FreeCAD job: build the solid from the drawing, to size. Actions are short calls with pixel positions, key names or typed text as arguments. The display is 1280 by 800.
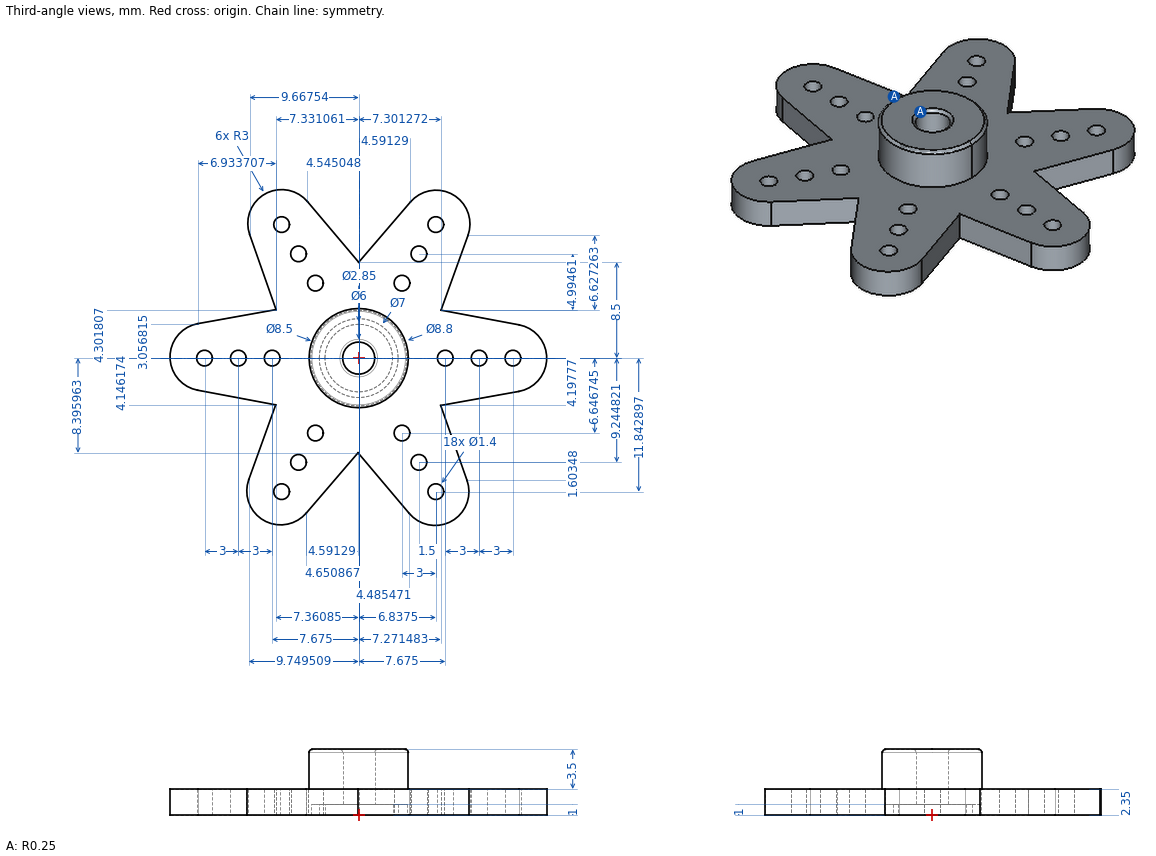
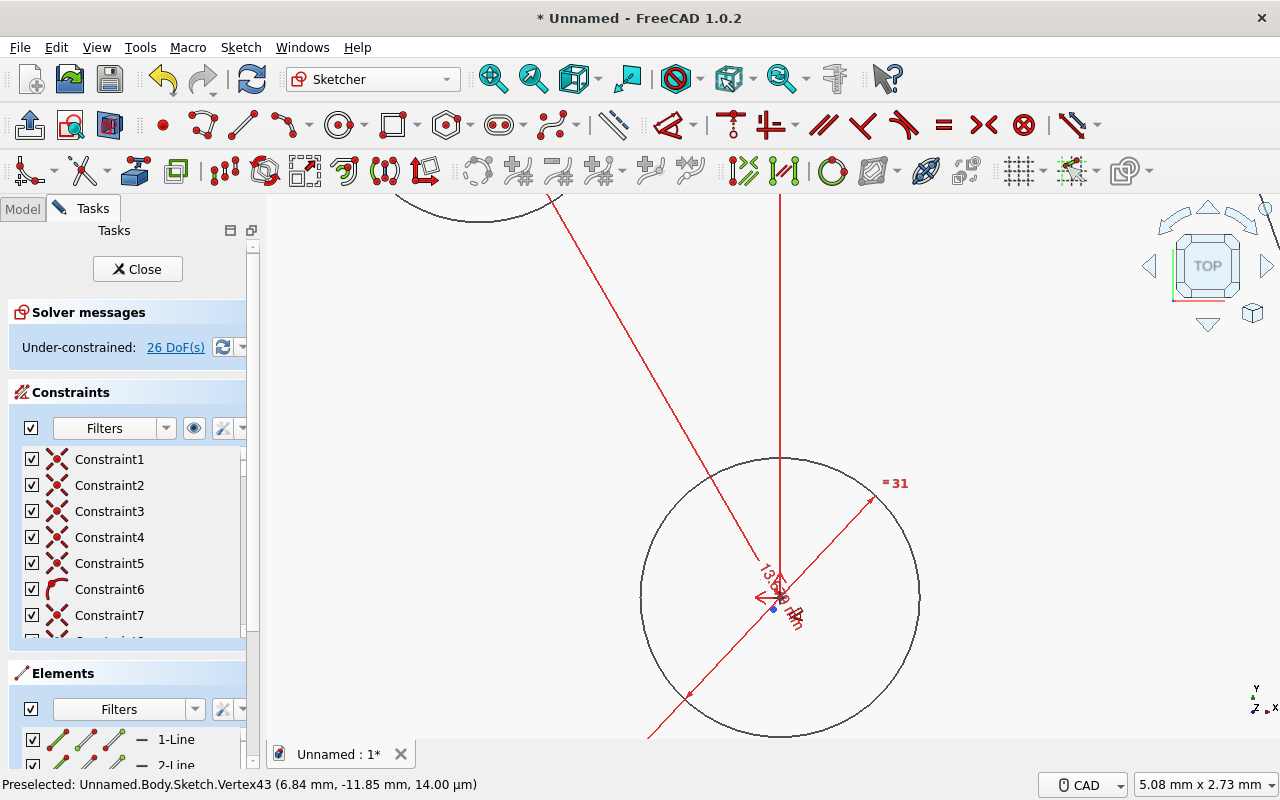
scroll(788, 612, down, 14)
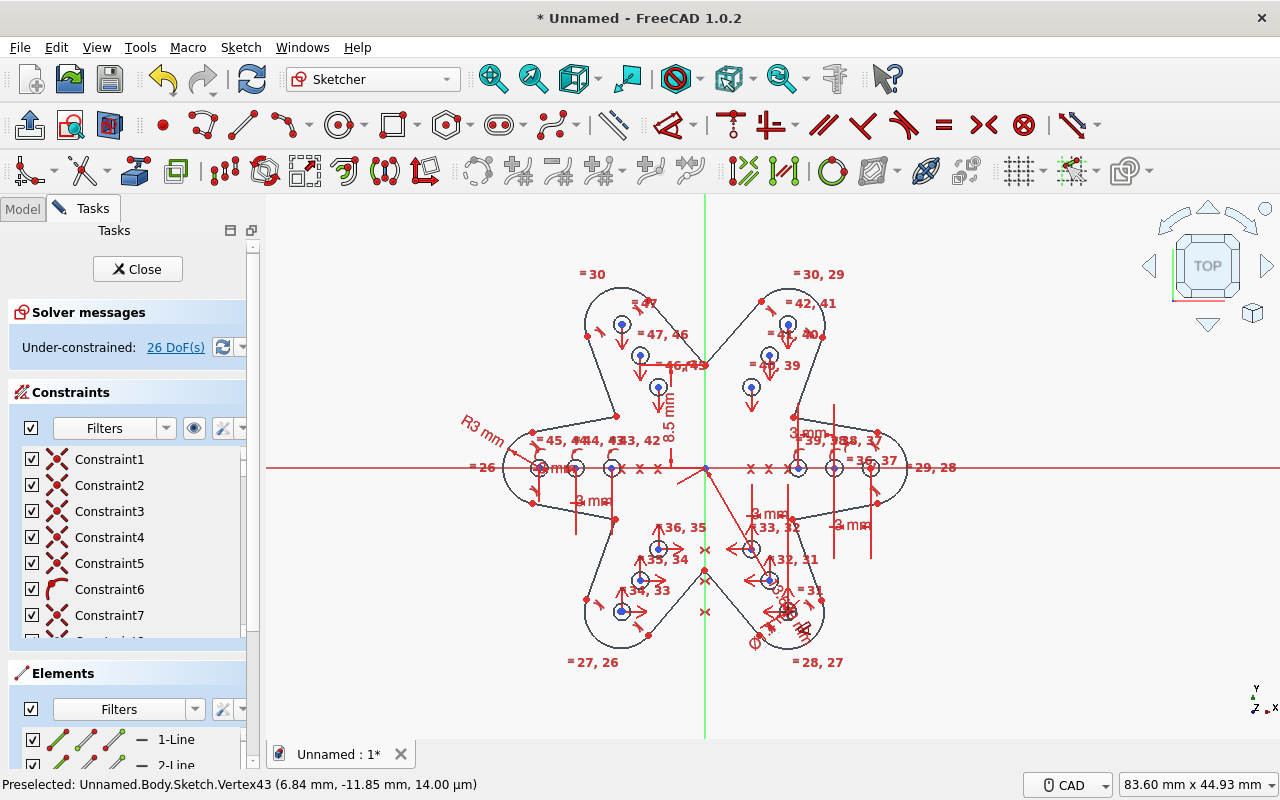
scroll(770, 581, up, 4)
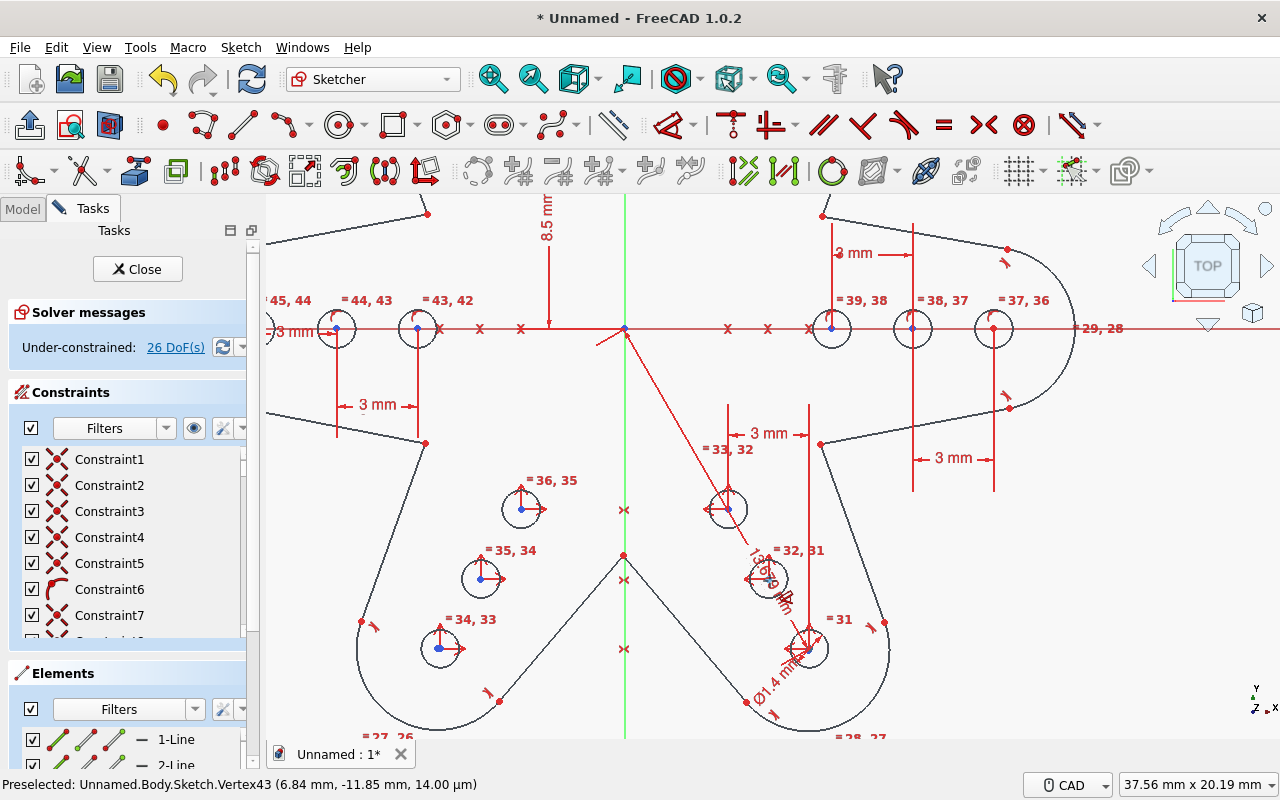
click(769, 579)
click(789, 545)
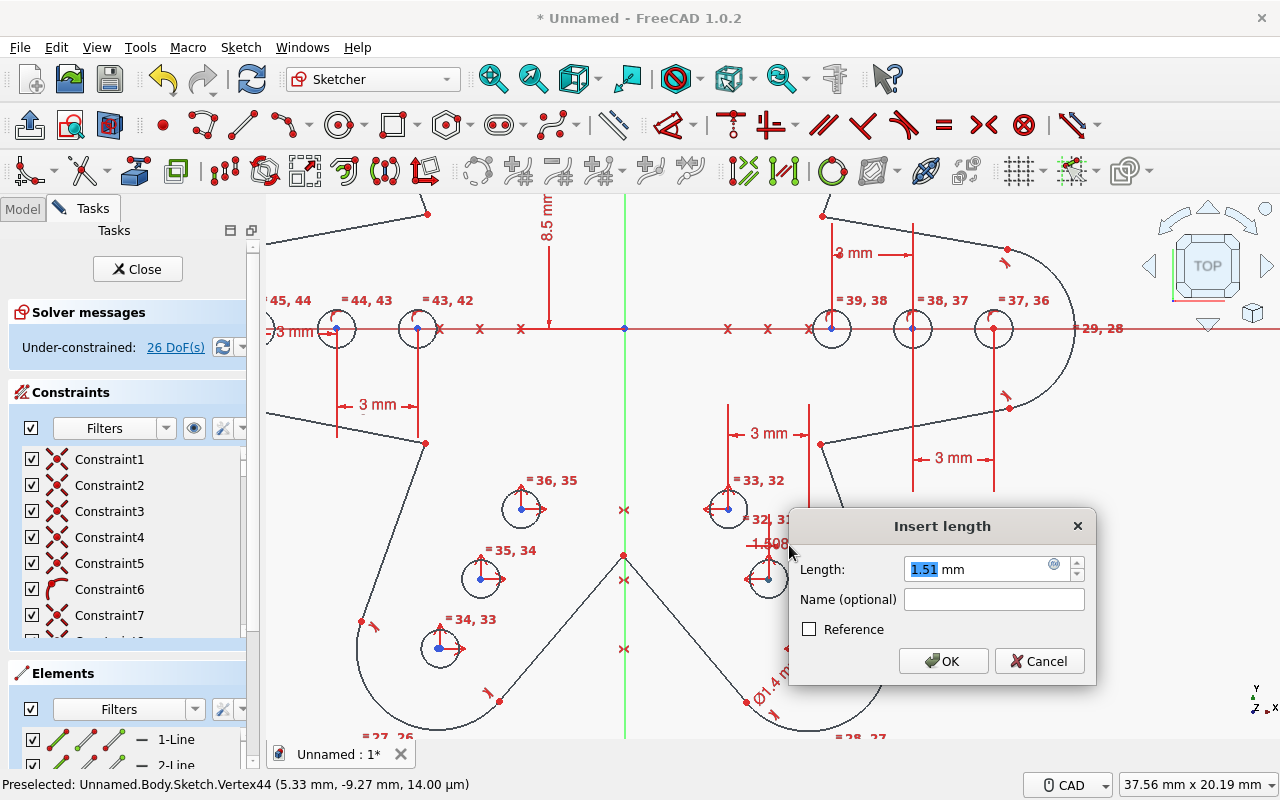
text(1.5)
key(Return)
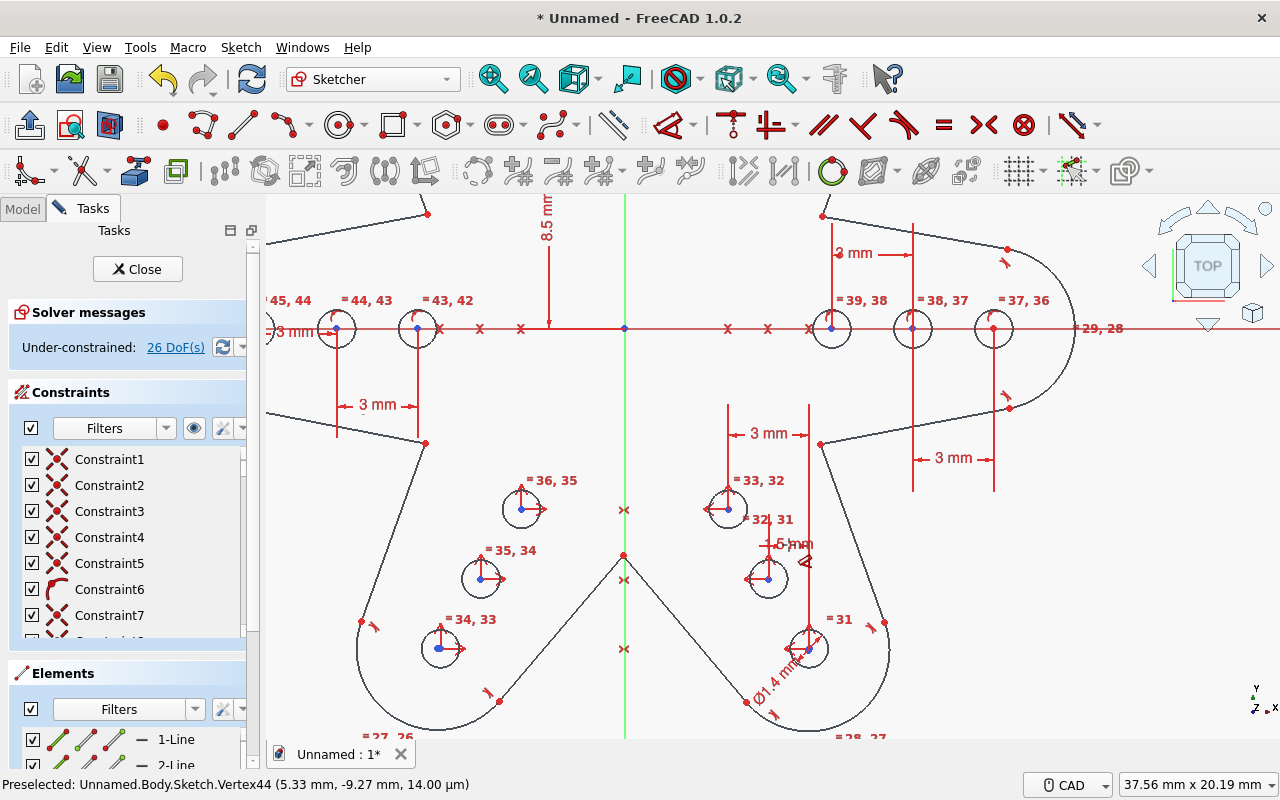
click(832, 329)
click(728, 363)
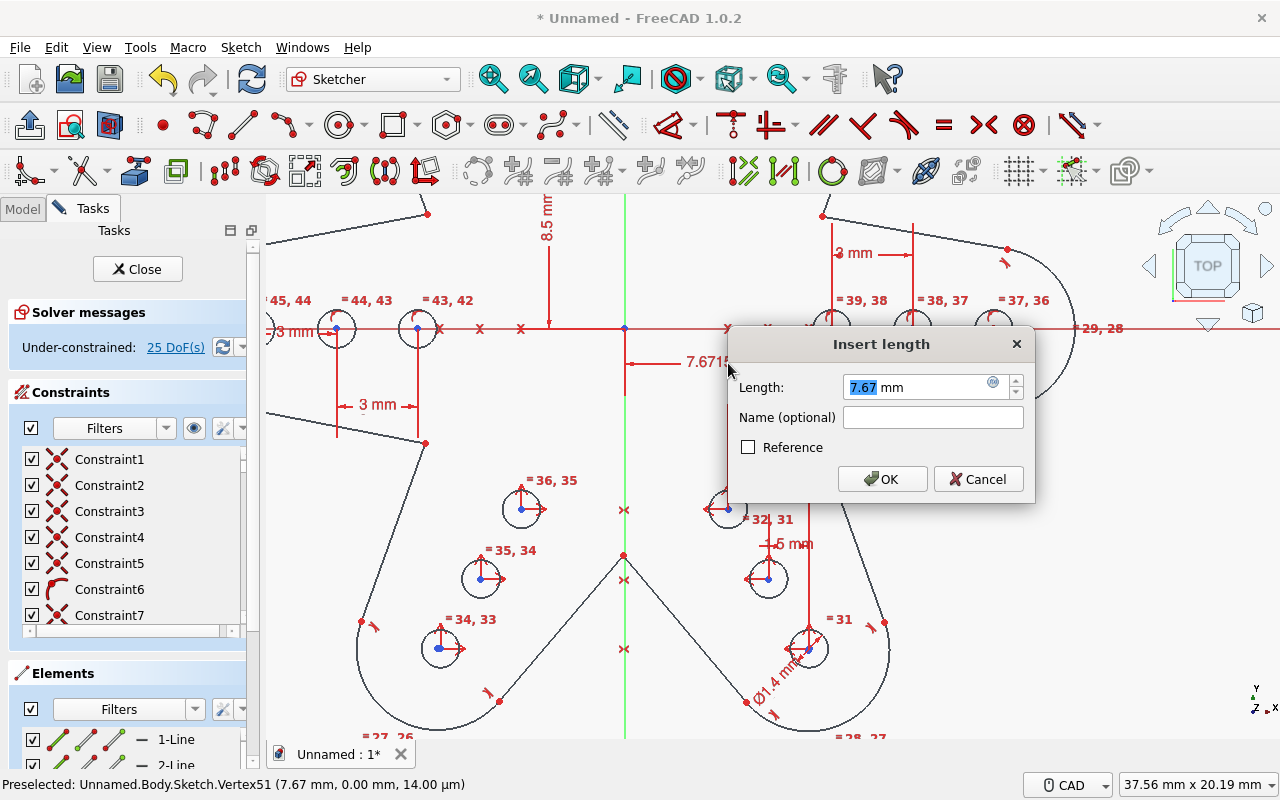
text(7.675)
key(Return)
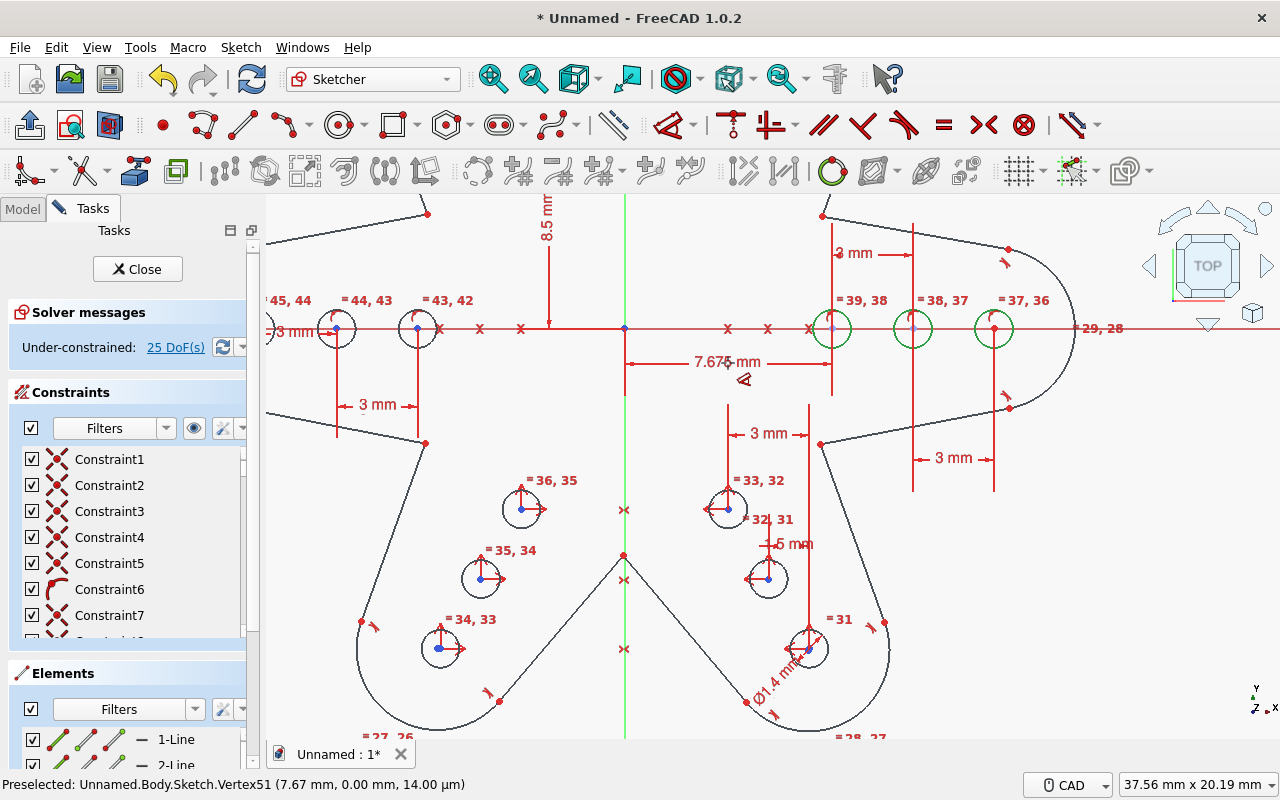
click(418, 329)
click(521, 363)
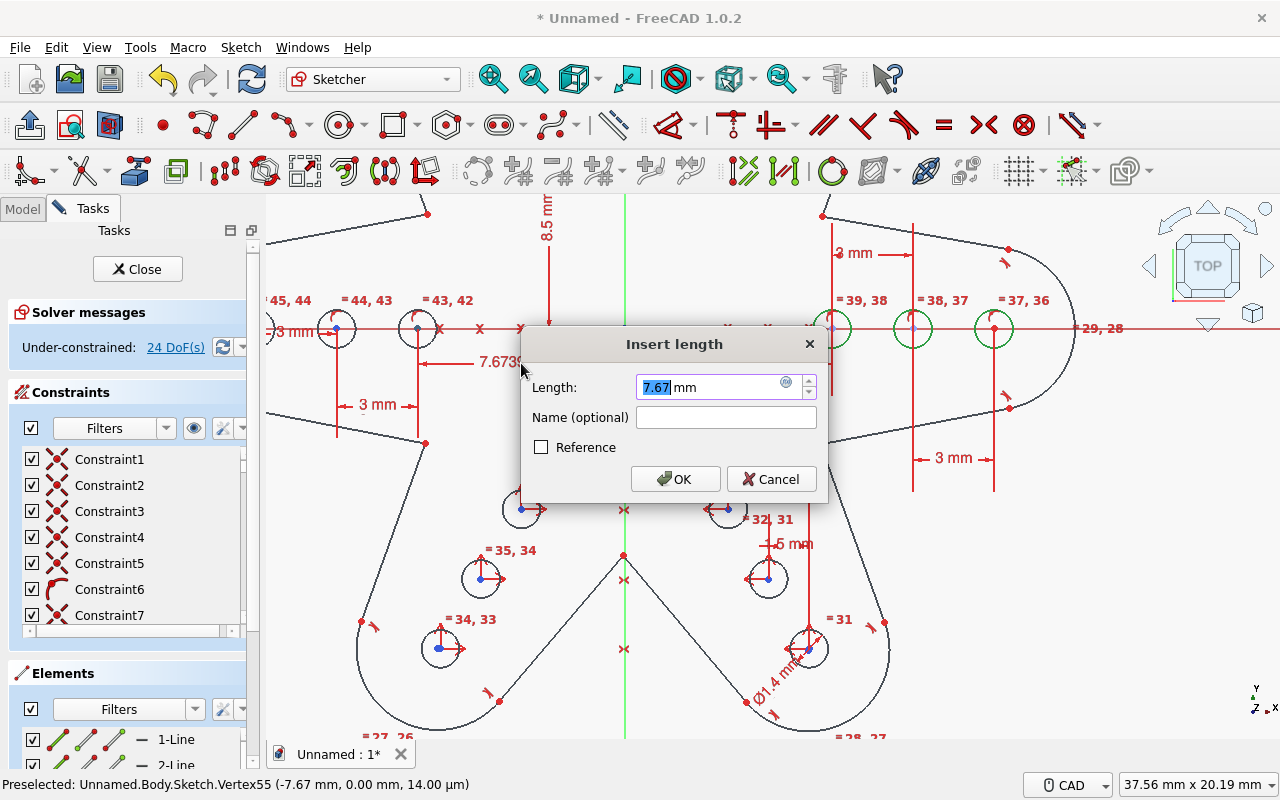
text(7.675)
key(Return)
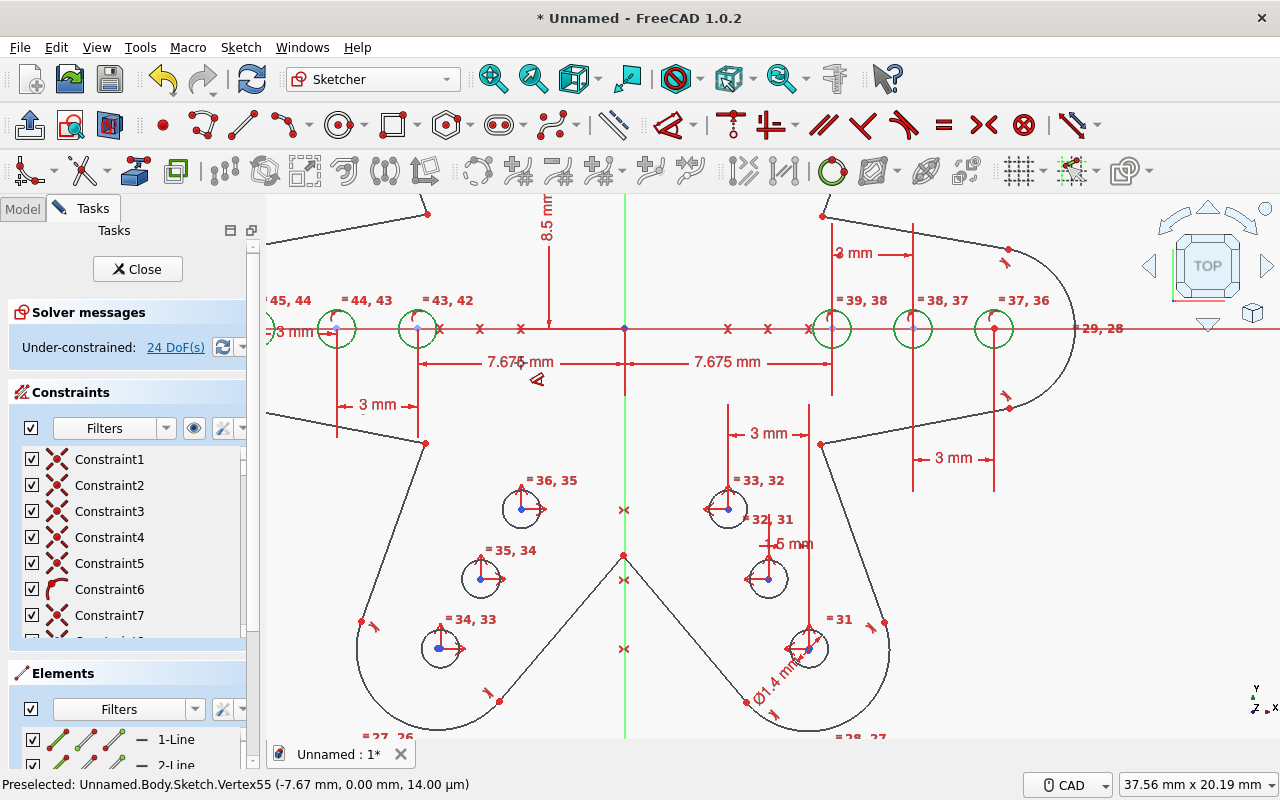
scroll(809, 649, up, 10)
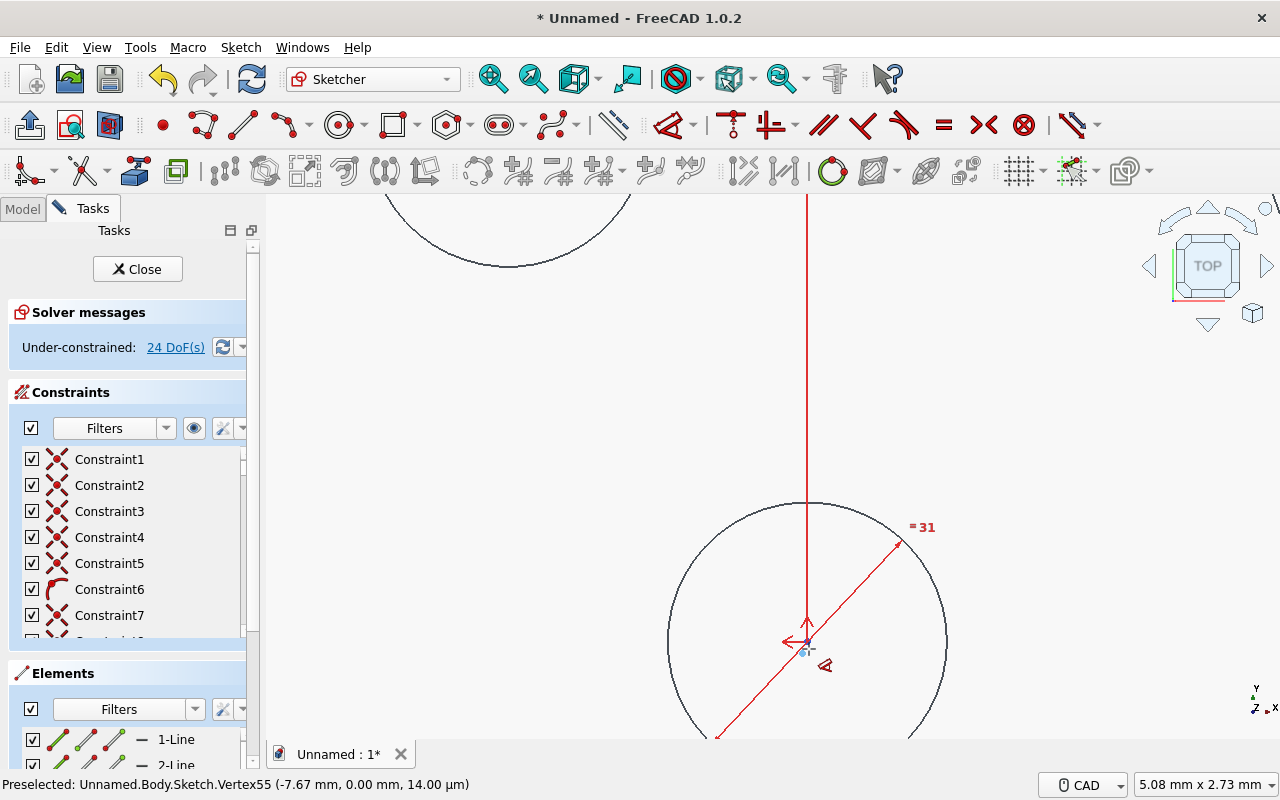
click(807, 642)
click(551, 676)